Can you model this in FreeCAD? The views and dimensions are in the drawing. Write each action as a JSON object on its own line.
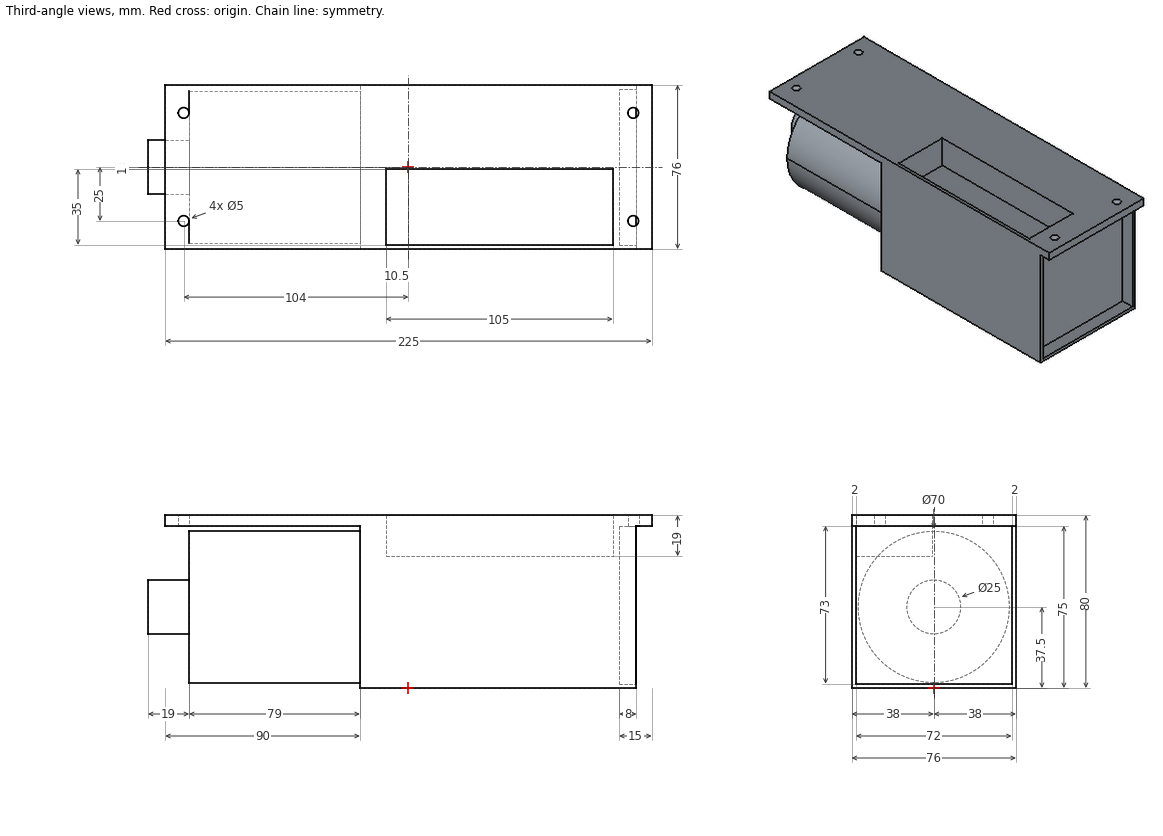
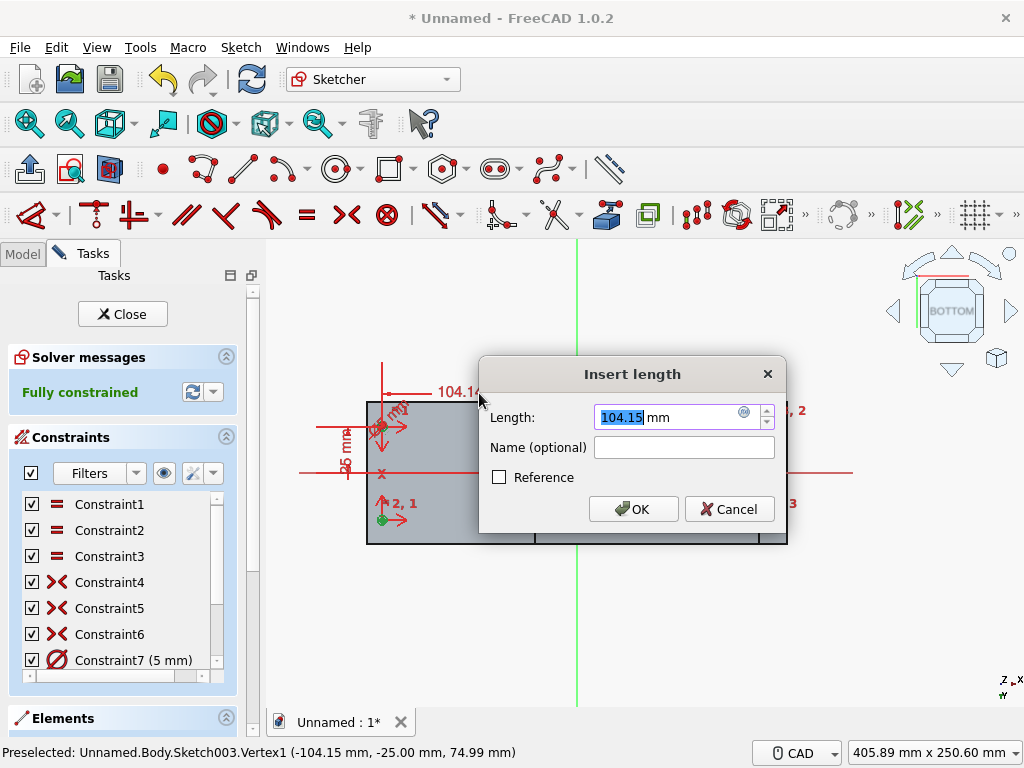
{"action": "type", "text": "104"}
{"action": "key", "text": "Return"}
{"action": "key", "text": "Escape"}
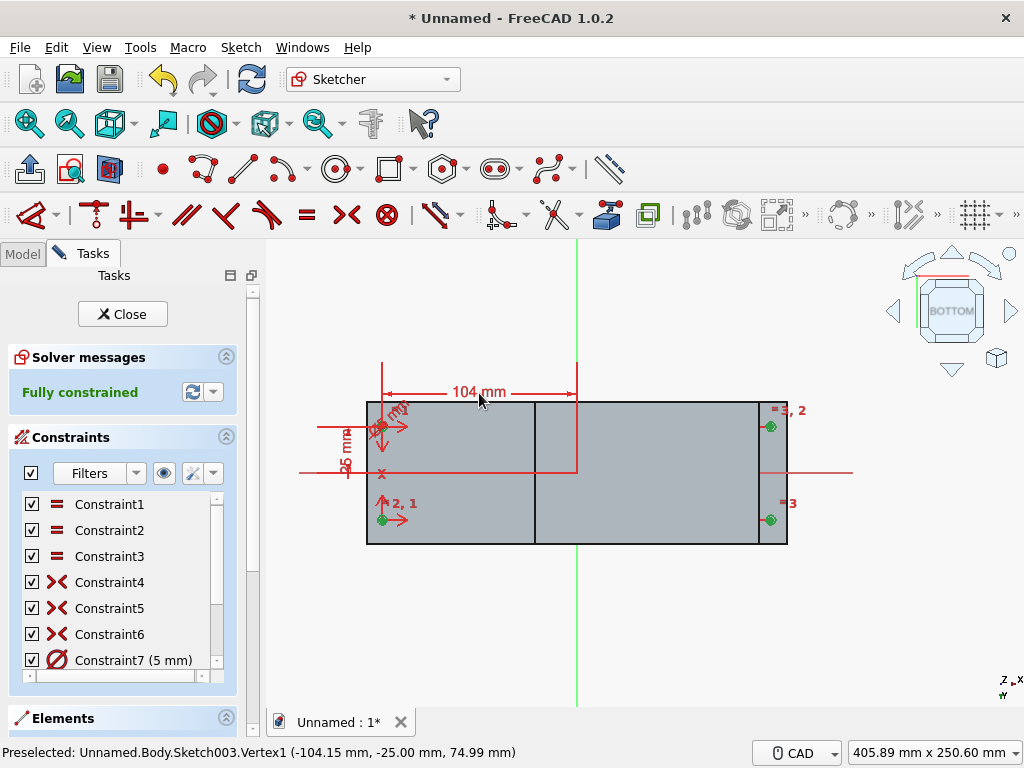
{"action": "left_click", "coordinate": [123, 314]}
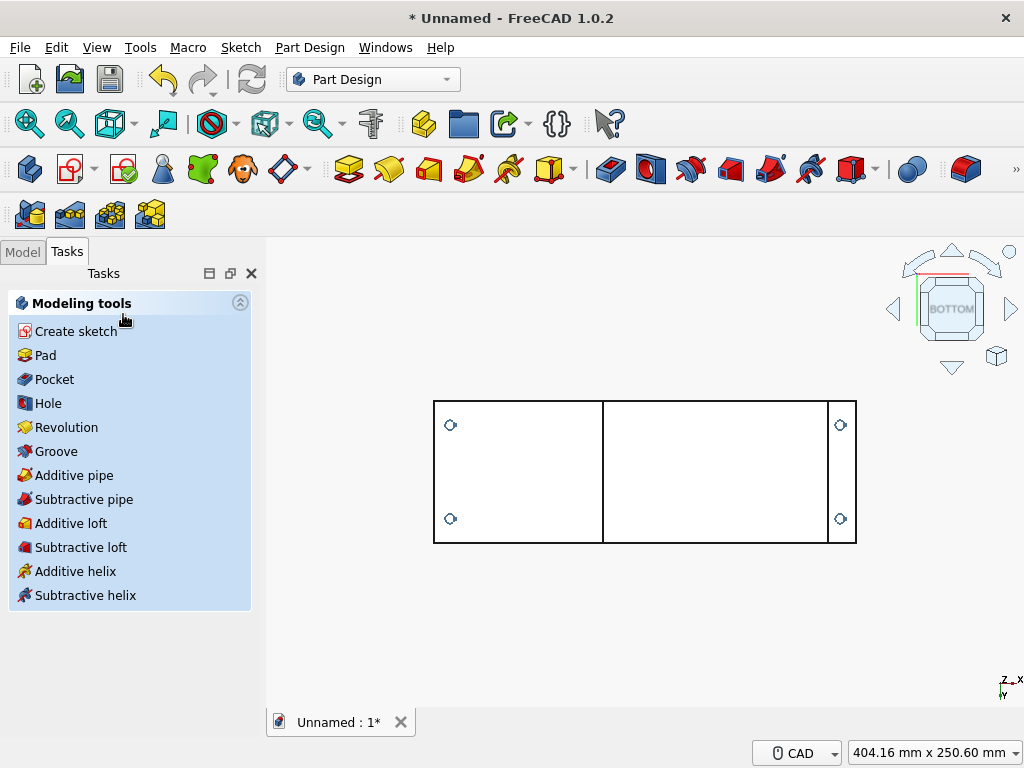
{"action": "left_click", "coordinate": [612, 170]}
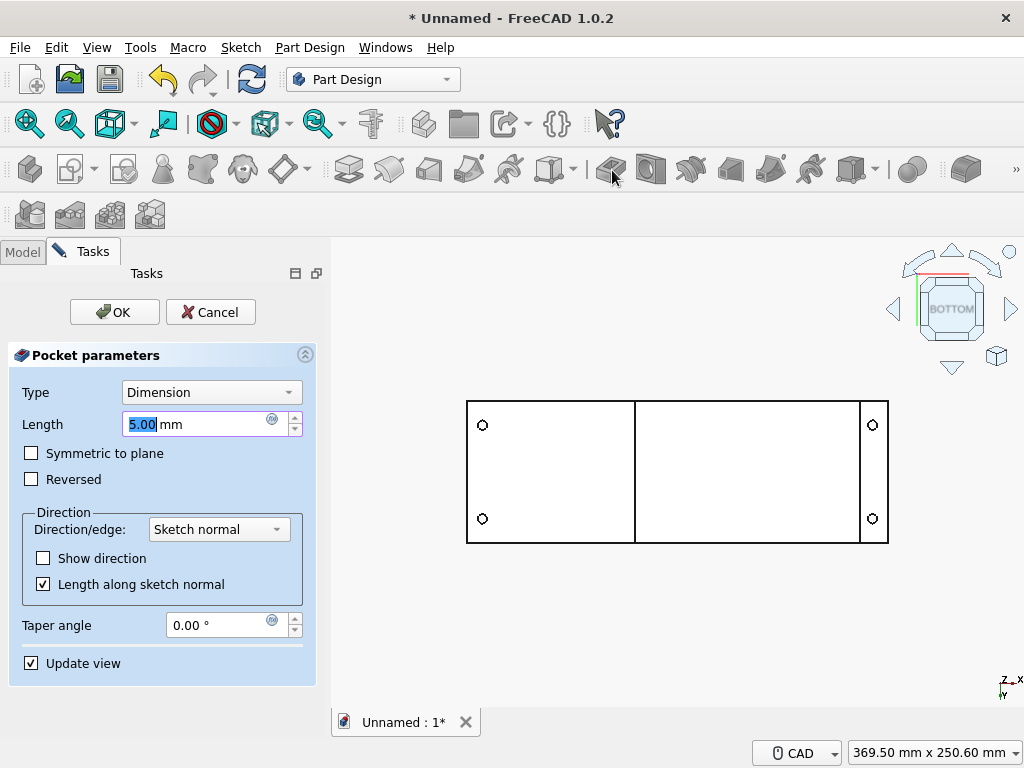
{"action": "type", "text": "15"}
{"action": "key", "text": "Tab"}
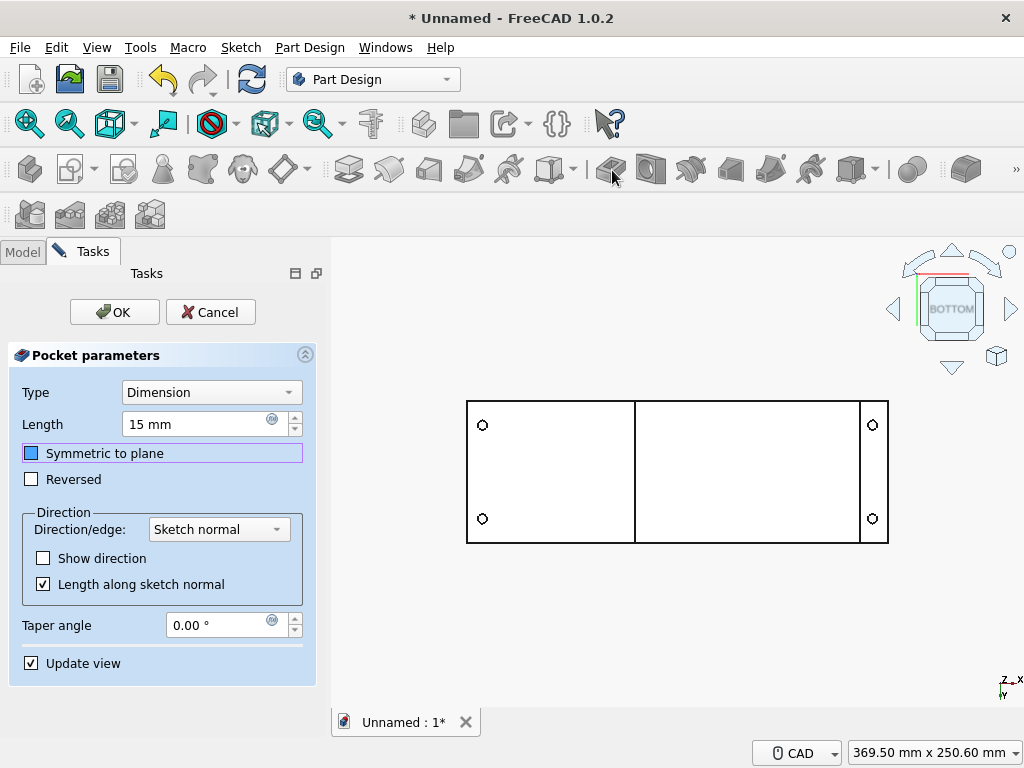
{"action": "left_click", "coordinate": [115, 312]}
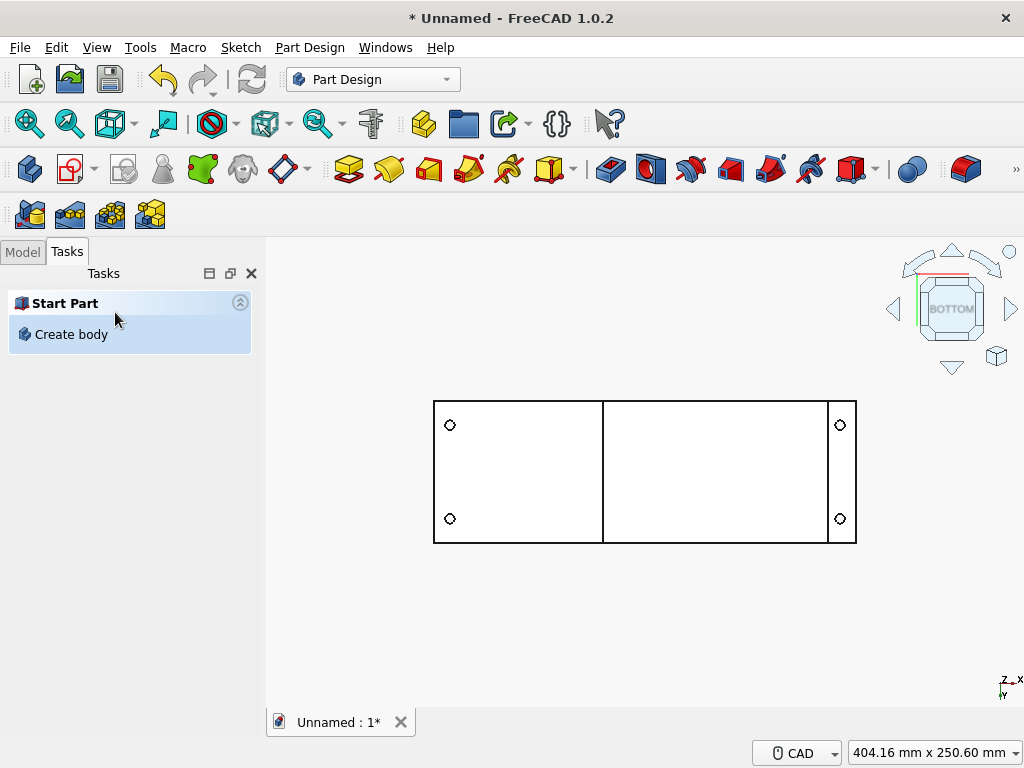
{"action": "key", "text": "6"}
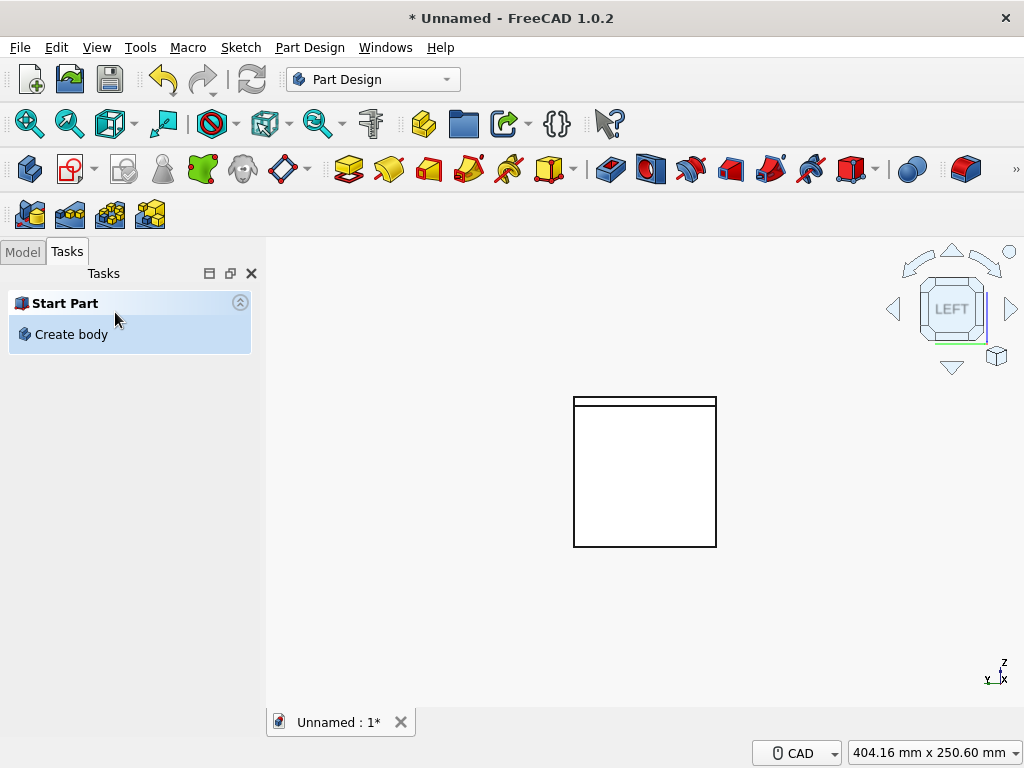
{"action": "key", "text": "v f"}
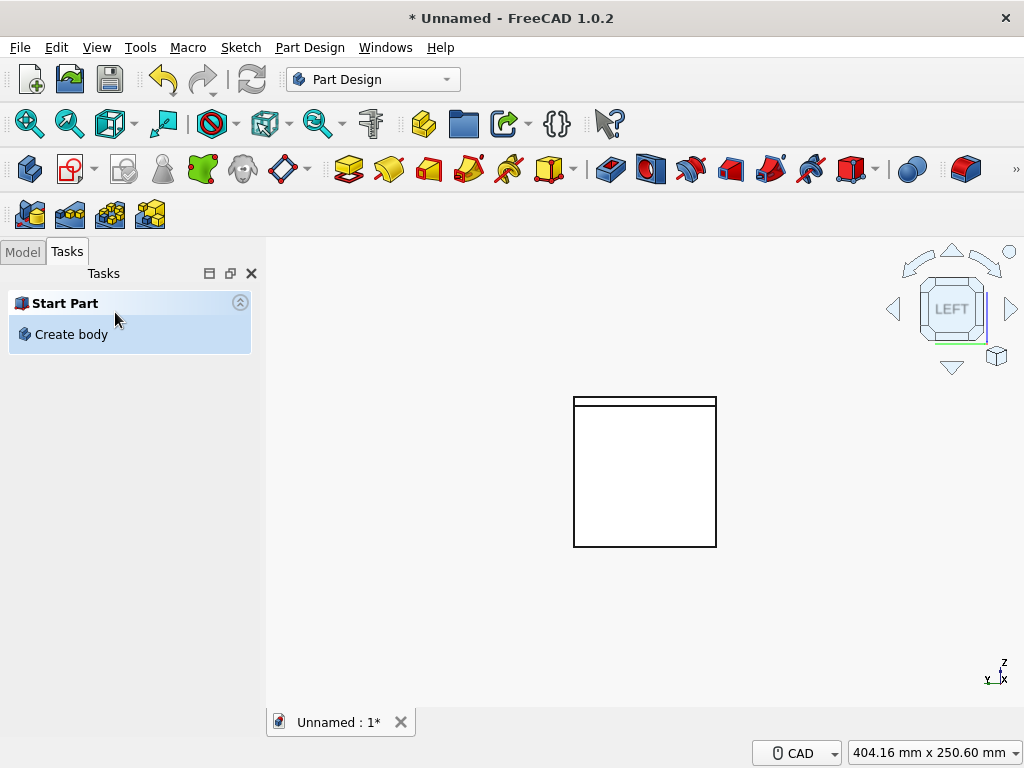
{"action": "left_click", "coordinate": [645, 476]}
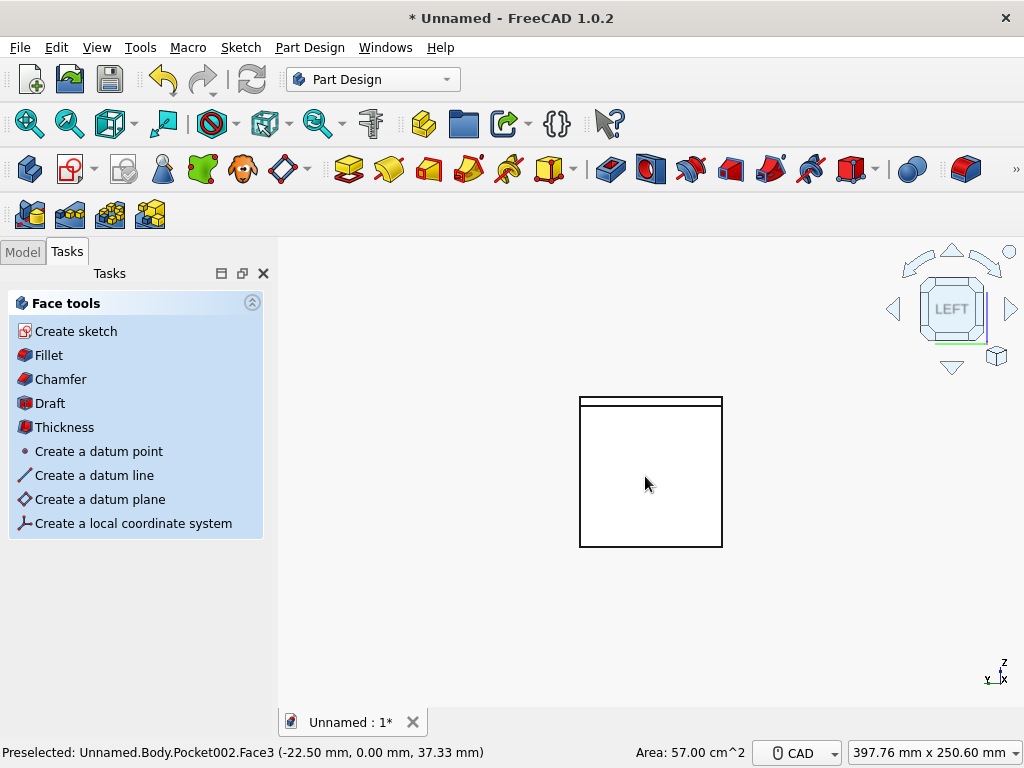
{"action": "left_click", "coordinate": [70, 170]}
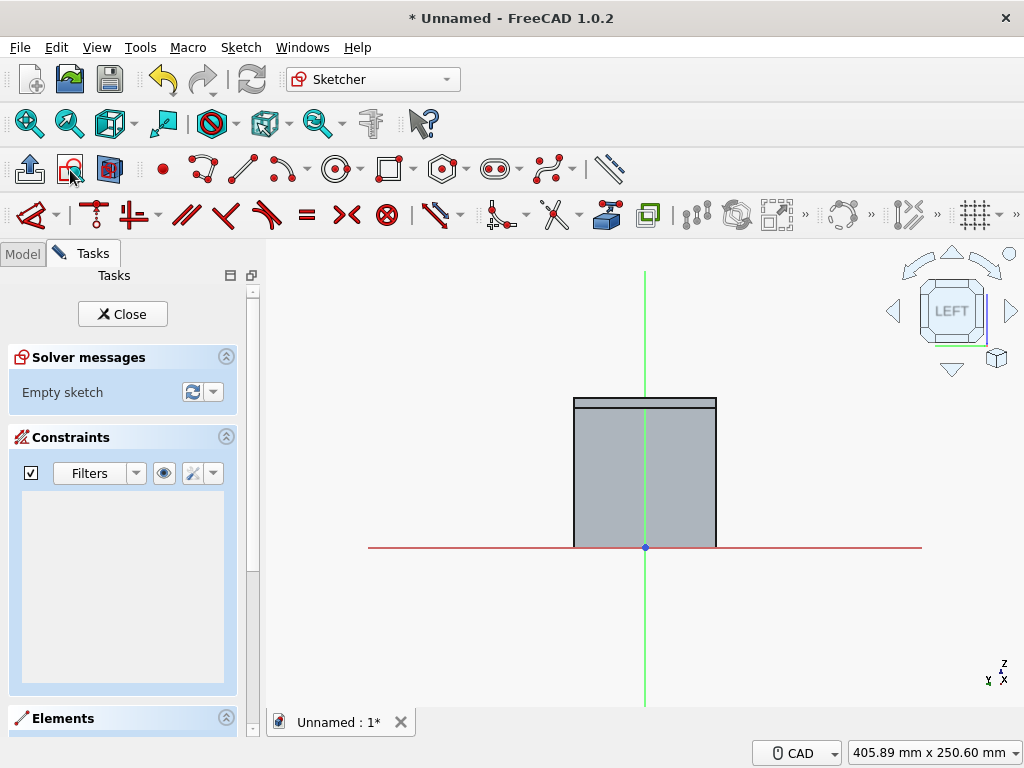
{"action": "key", "text": "q s"}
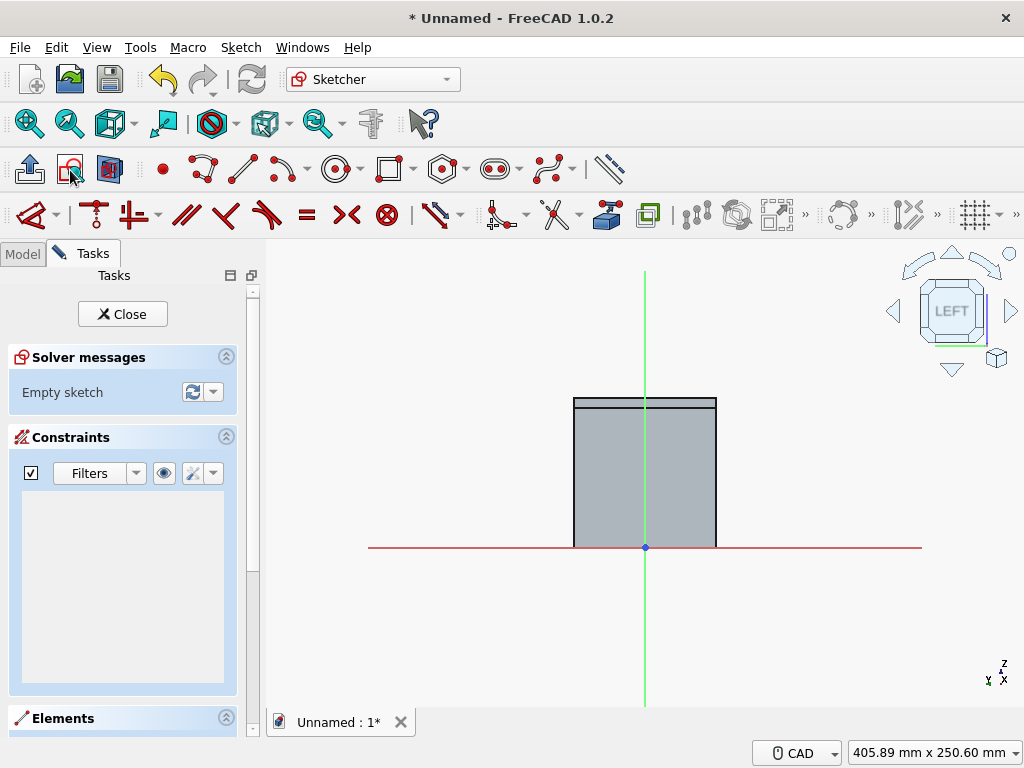
{"action": "scroll", "coordinate": [701, 486], "scroll_direction": "up", "scroll_amount": 4}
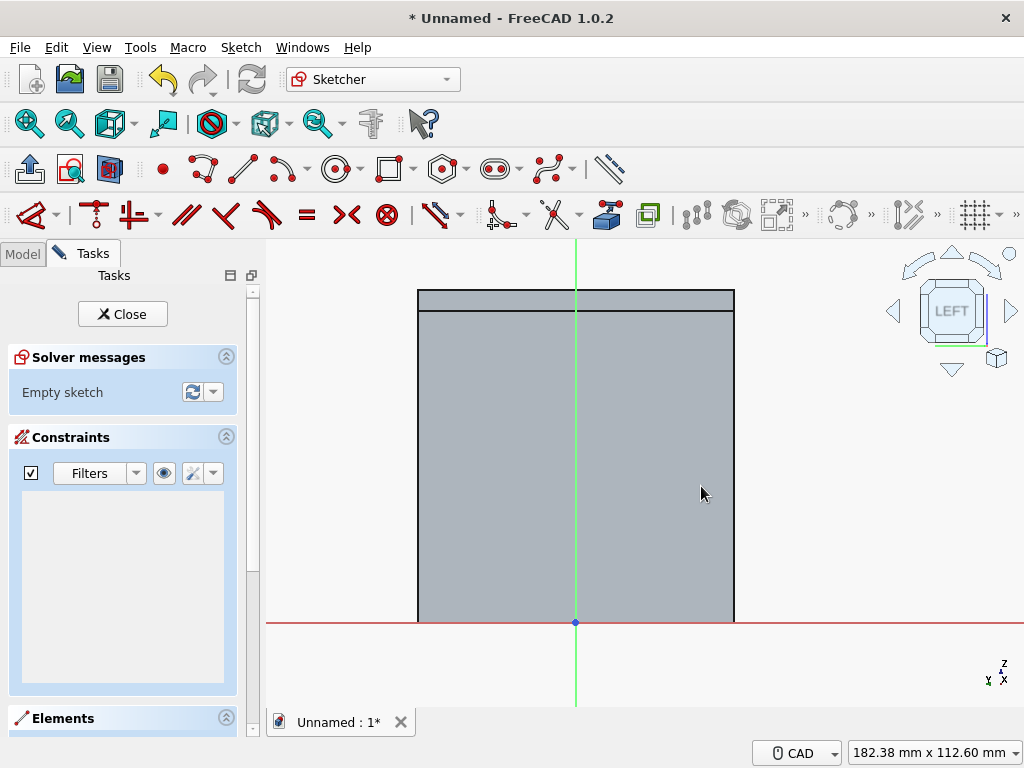
{"action": "key", "text": "g c"}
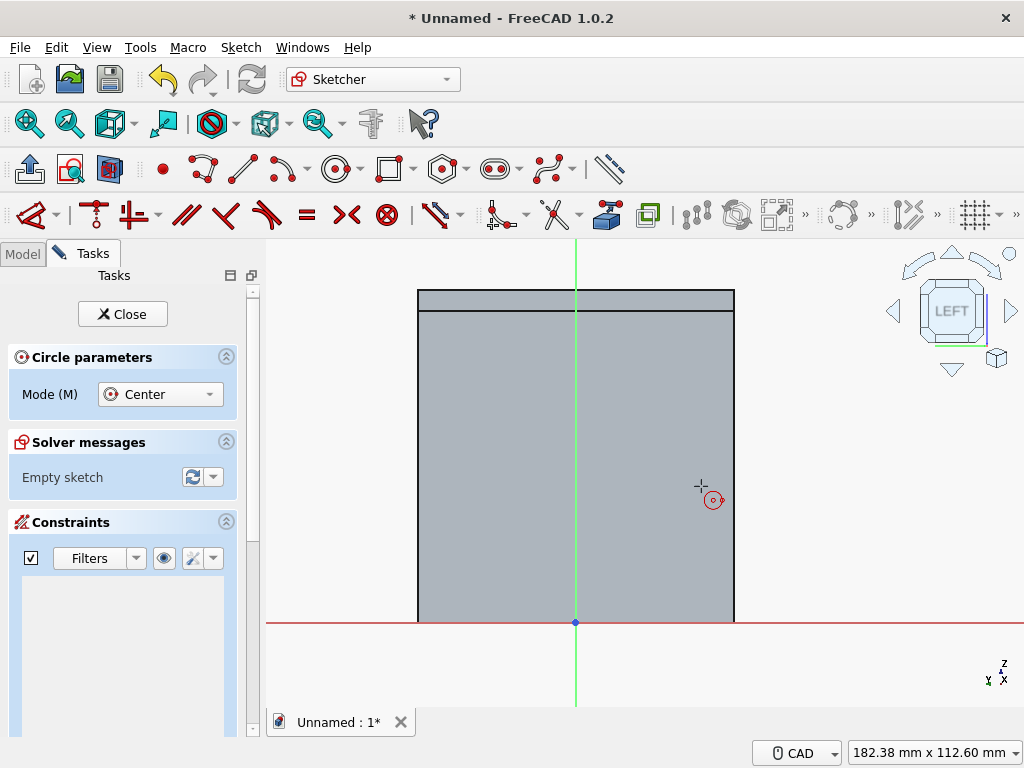
{"action": "left_click", "coordinate": [576, 467]}
{"action": "left_click", "coordinate": [679, 364]}
{"action": "key", "text": "Escape"}